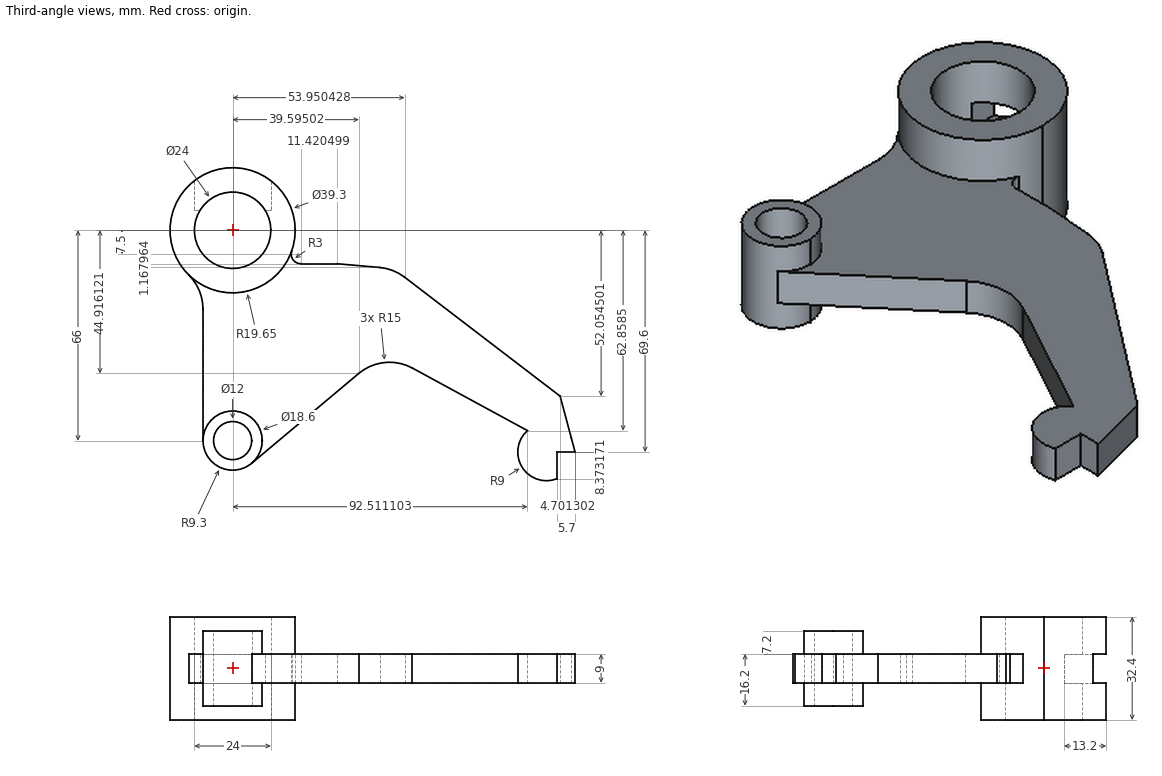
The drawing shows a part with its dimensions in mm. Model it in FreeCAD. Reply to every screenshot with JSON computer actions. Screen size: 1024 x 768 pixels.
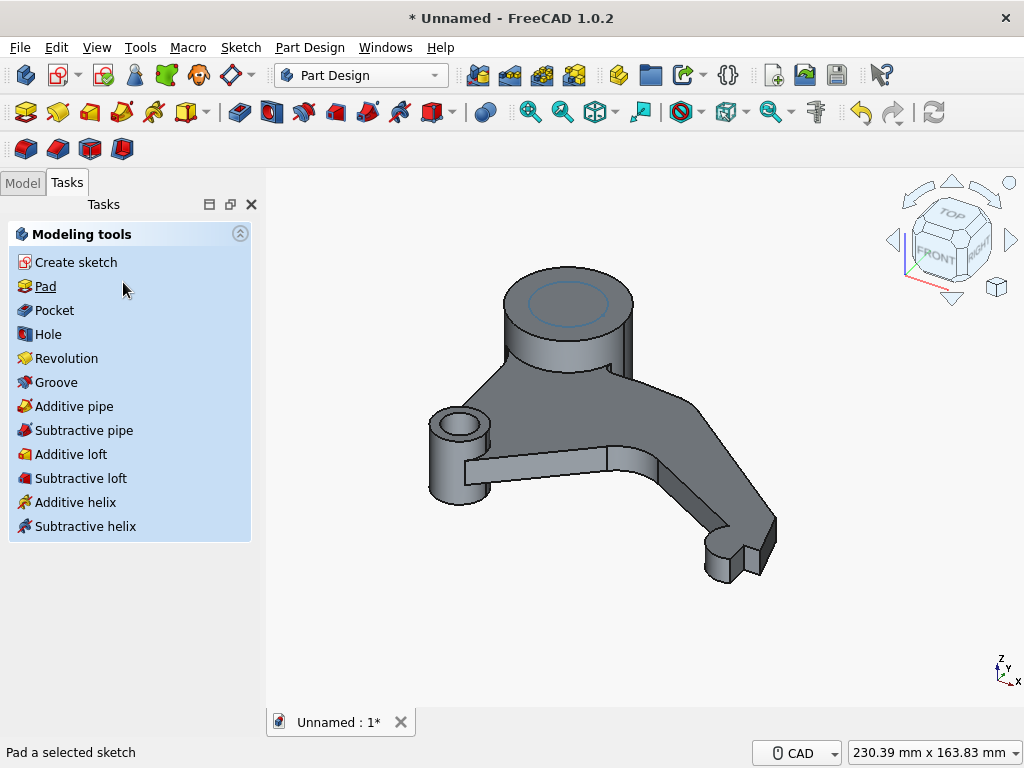
{"action": "left_click", "coordinate": [240, 112]}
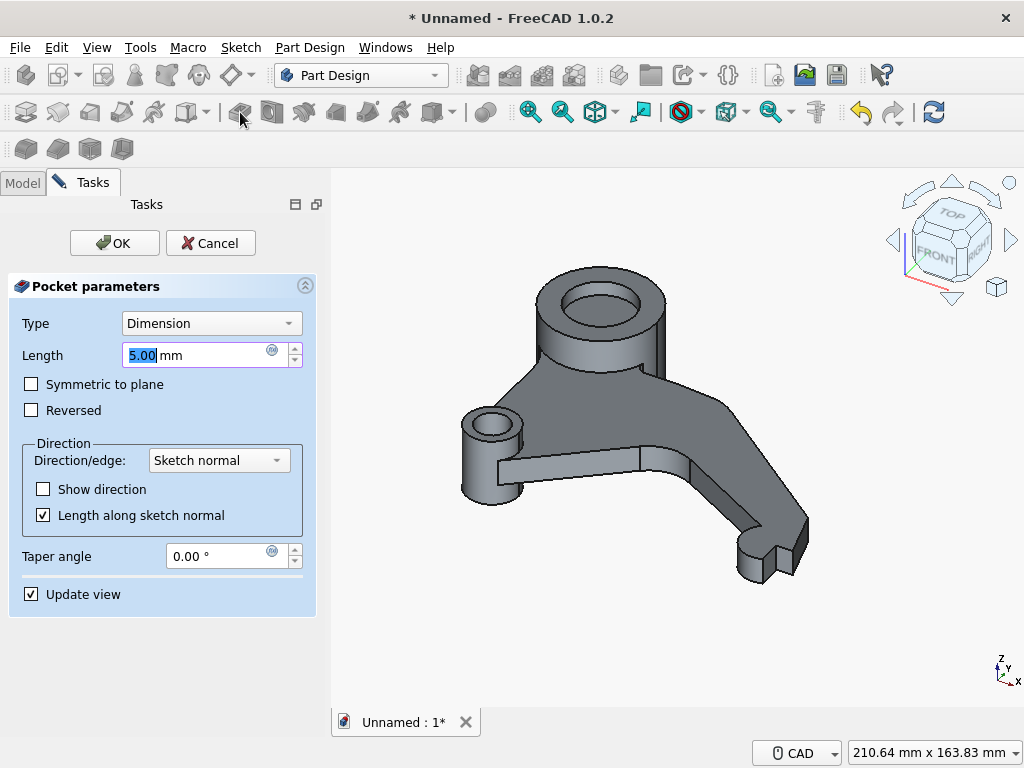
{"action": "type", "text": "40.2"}
{"action": "key", "text": "Tab"}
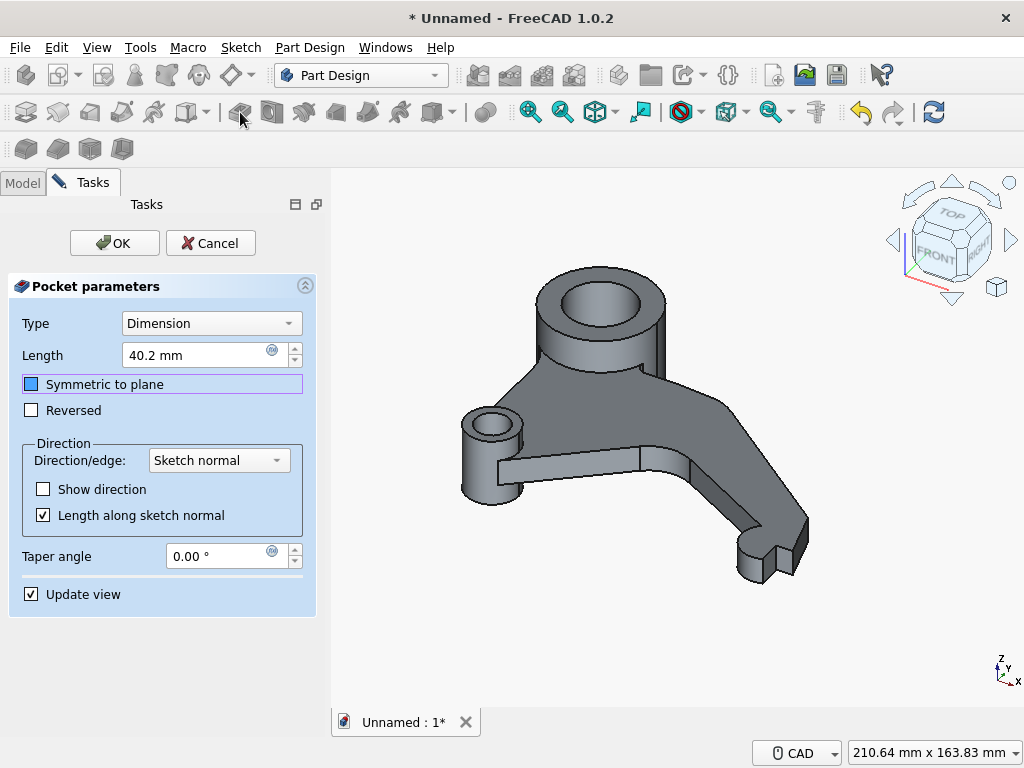
{"action": "left_click", "coordinate": [115, 243]}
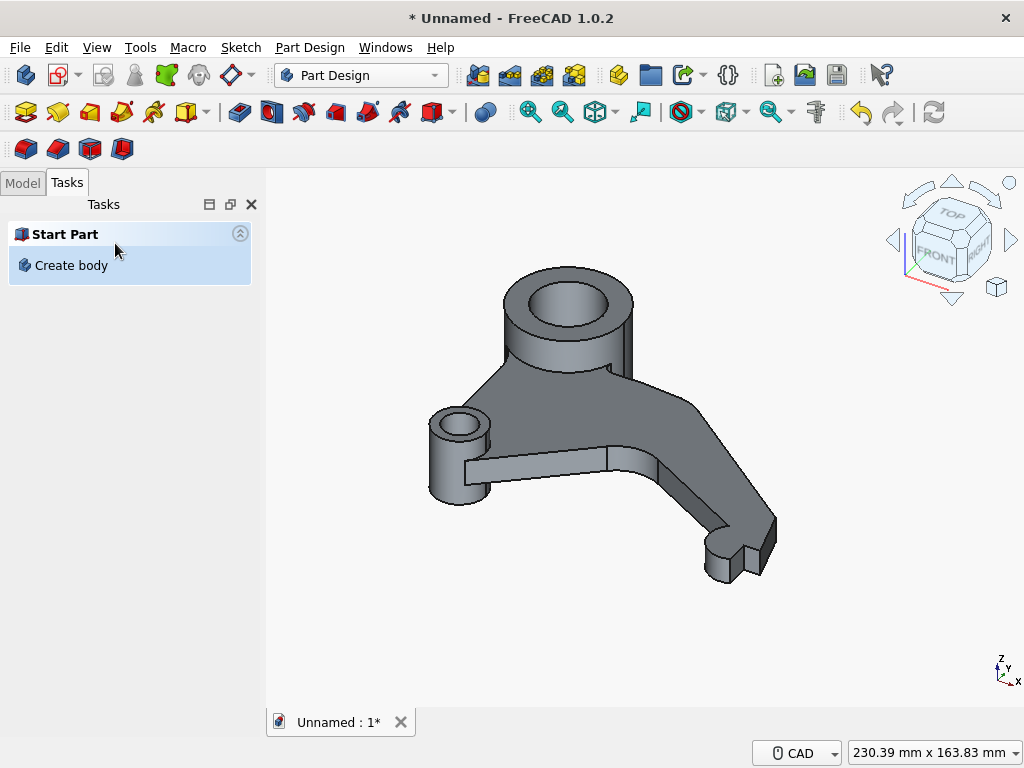
{"action": "left_click", "coordinate": [23, 182]}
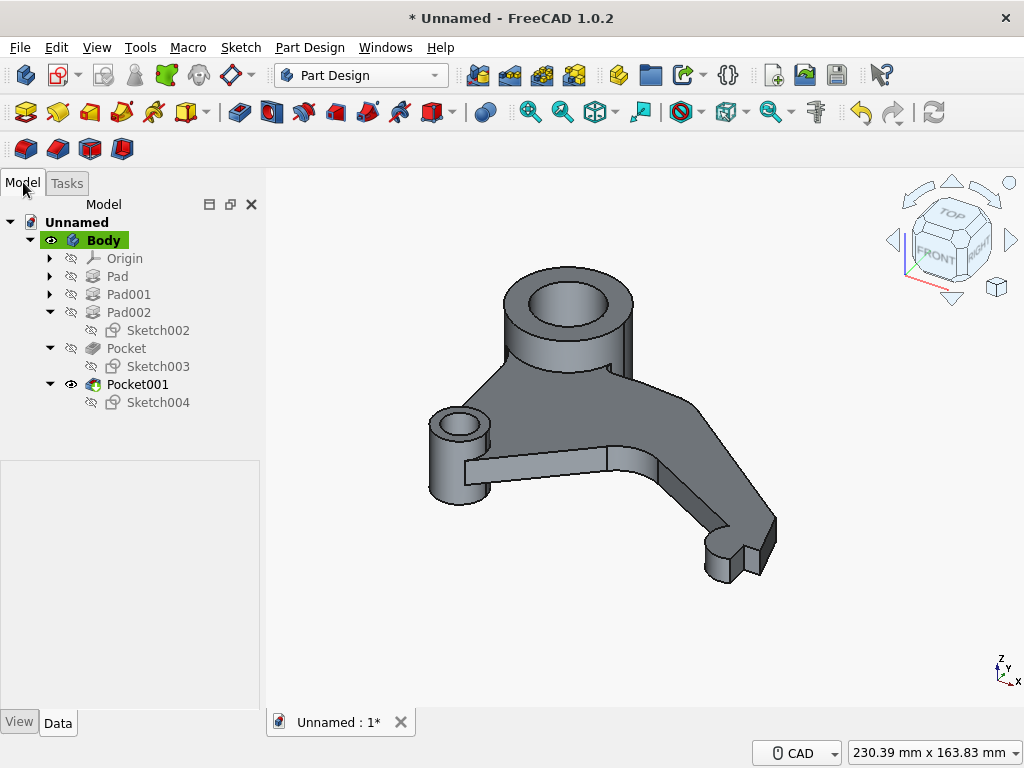
{"action": "left_click", "coordinate": [50, 258]}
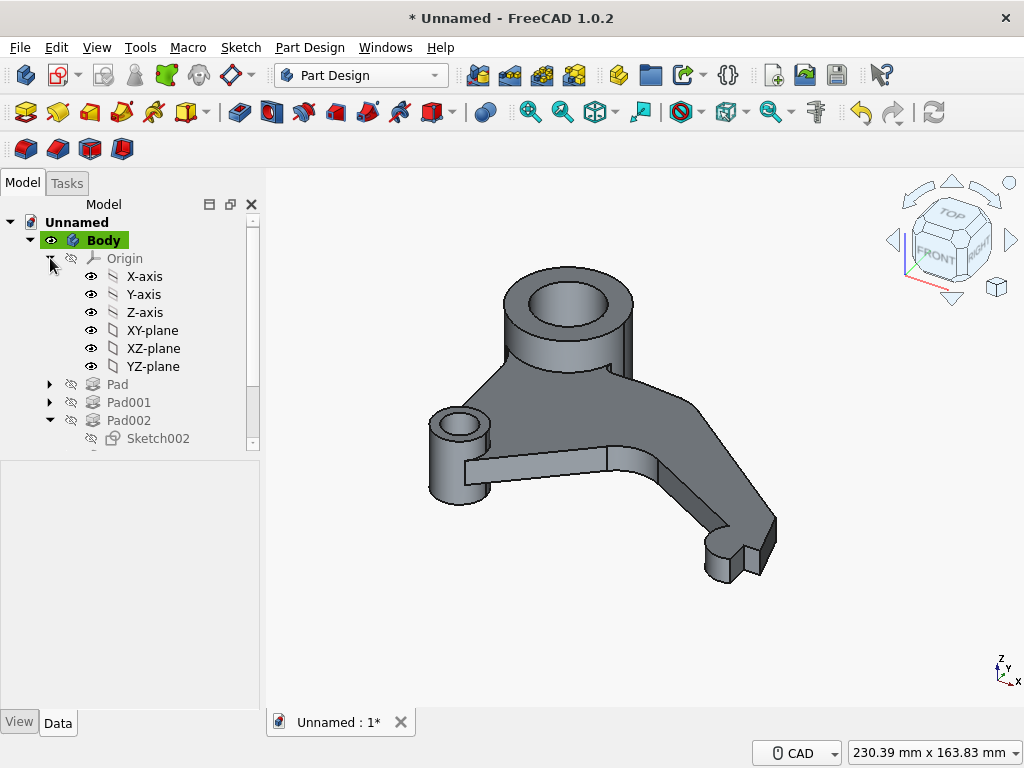
{"action": "left_click", "coordinate": [136, 348]}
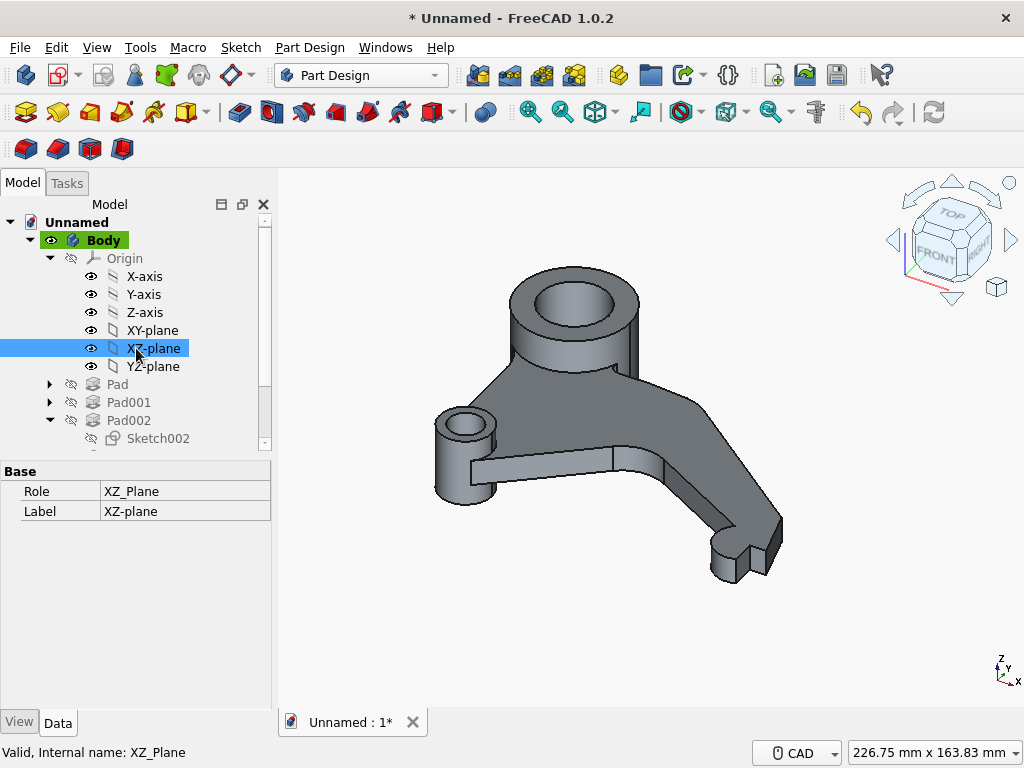
{"action": "left_click", "coordinate": [232, 76]}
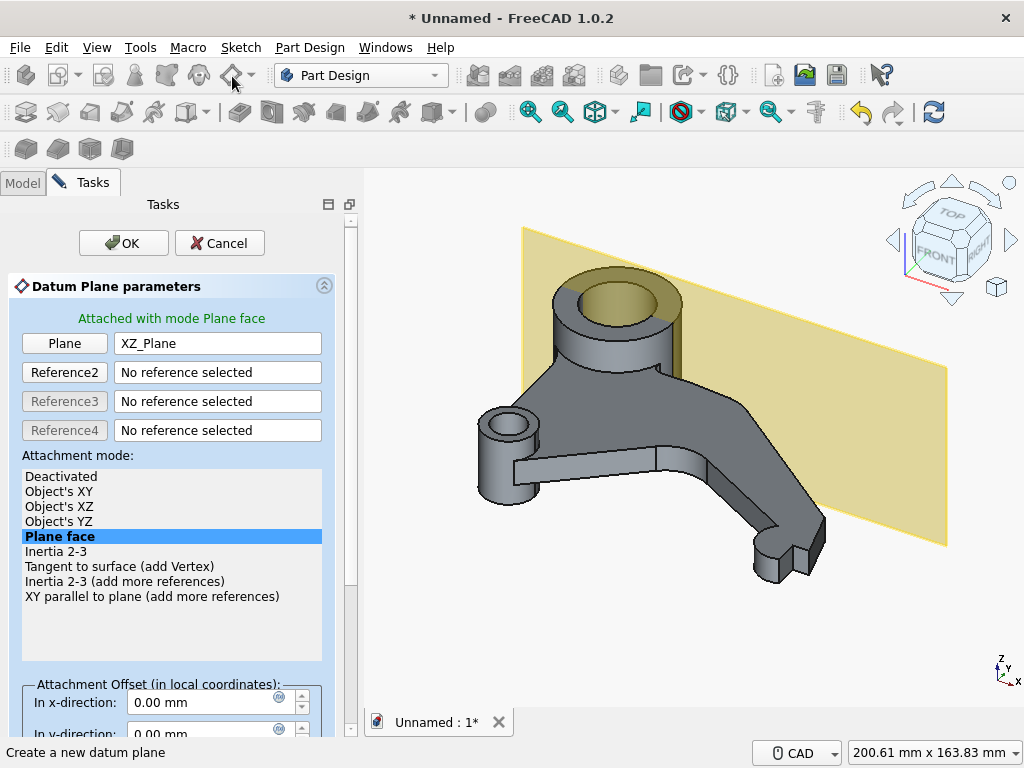
{"action": "scroll", "coordinate": [351, 475], "scroll_direction": "down", "scroll_amount": 2}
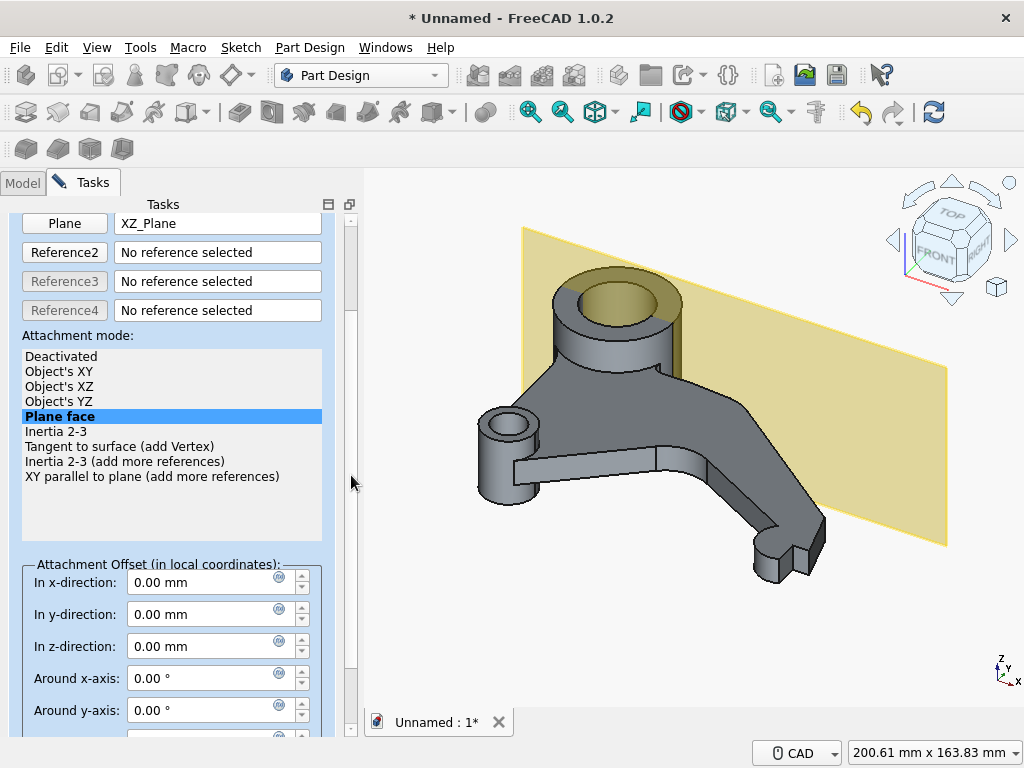
{"action": "triple_click", "coordinate": [210, 646]}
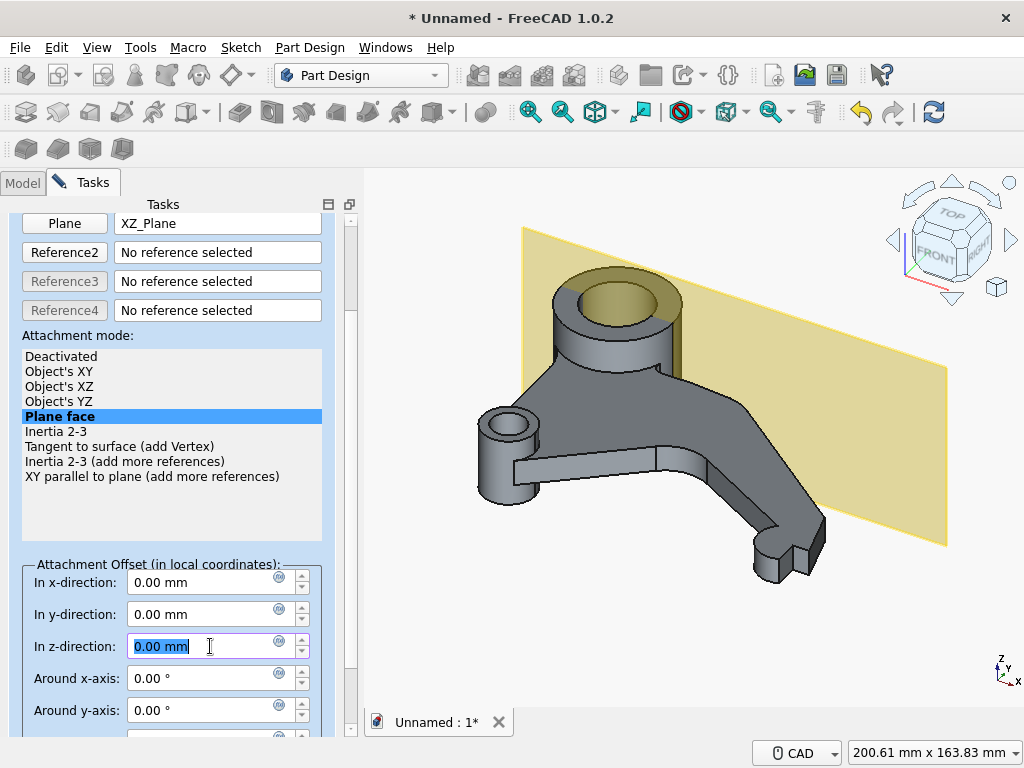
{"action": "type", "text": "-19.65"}
{"action": "key", "text": "Tab"}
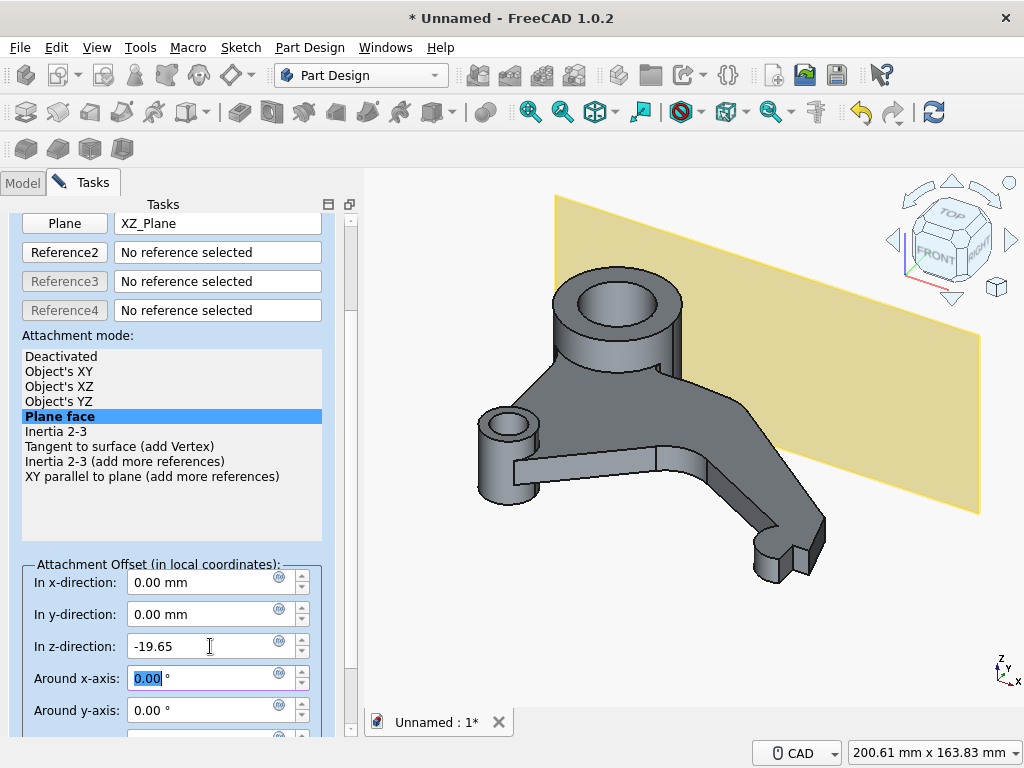
{"action": "scroll", "coordinate": [351, 475], "scroll_direction": "up", "scroll_amount": 3}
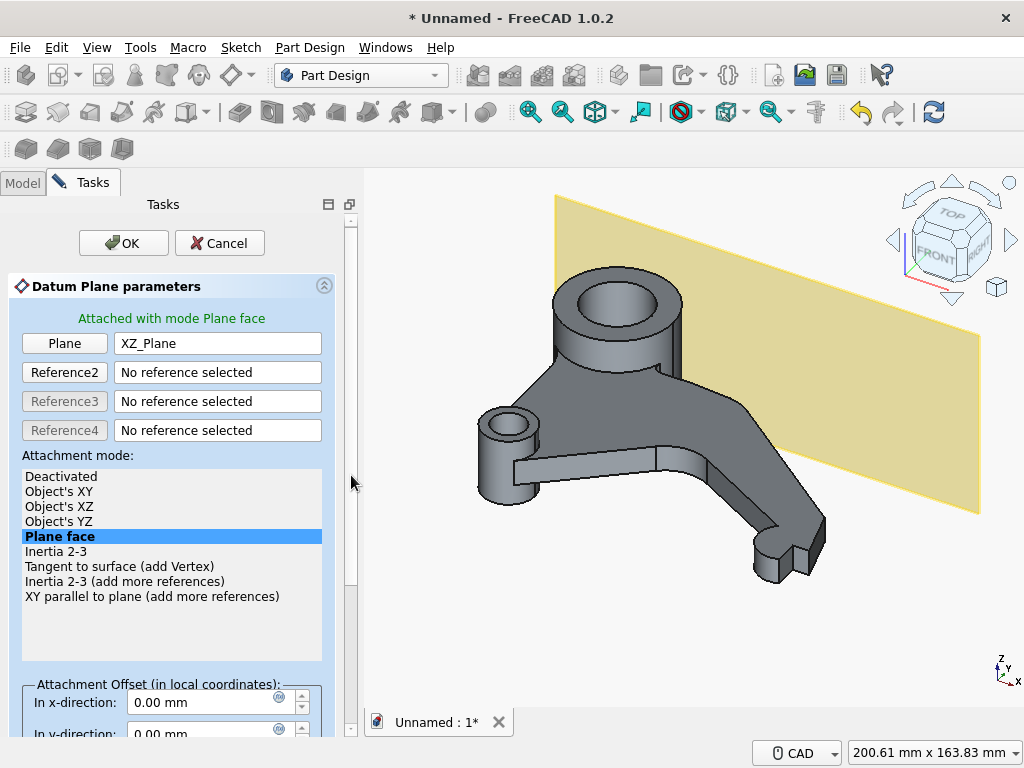
{"action": "left_click", "coordinate": [124, 243]}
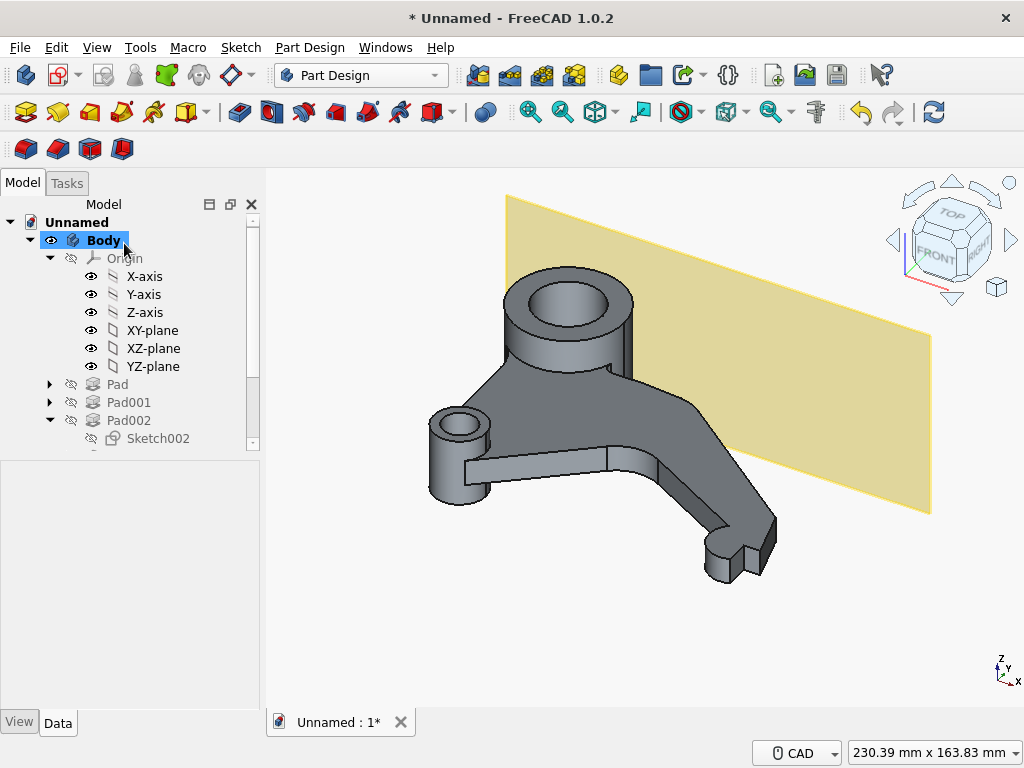
{"action": "scroll", "coordinate": [100, 326], "scroll_direction": "down", "scroll_amount": 3}